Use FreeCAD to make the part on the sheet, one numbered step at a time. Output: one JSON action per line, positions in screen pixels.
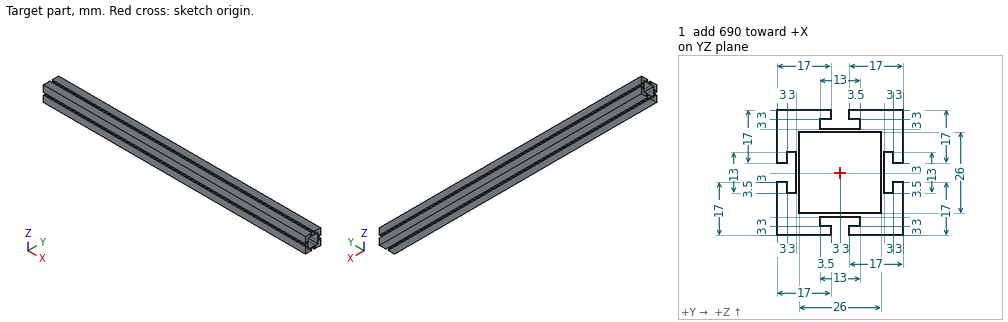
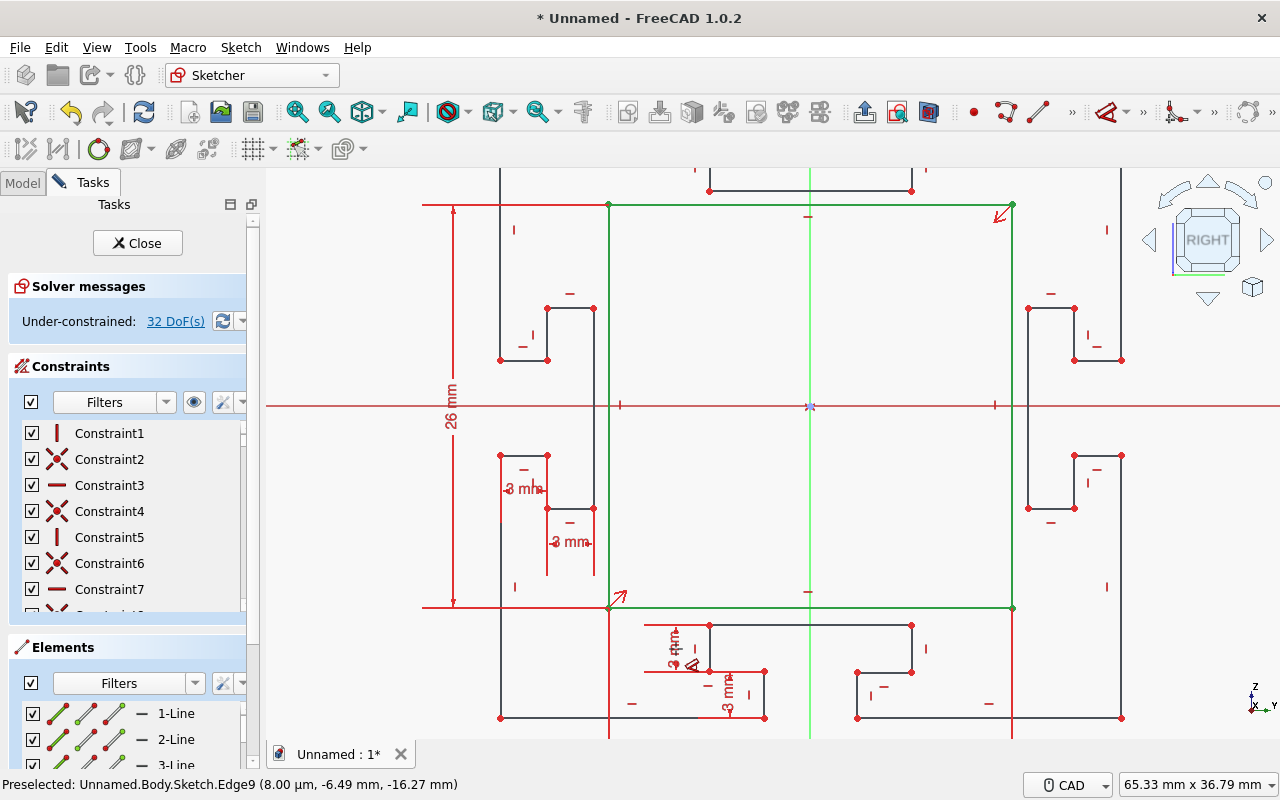
{"action": "left_click", "coordinate": [912, 639]}
{"action": "left_click", "coordinate": [946, 649]}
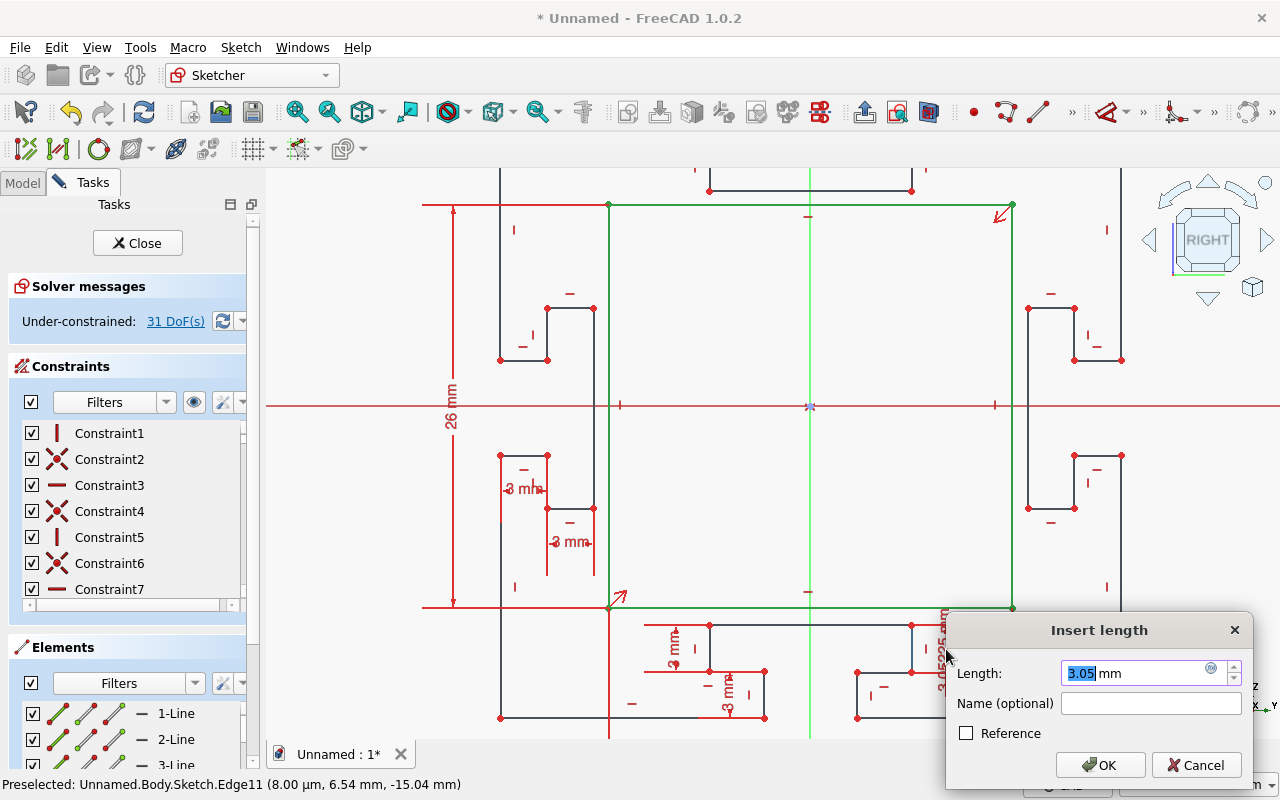
{"action": "type", "text": "3"}
{"action": "key", "text": "Return"}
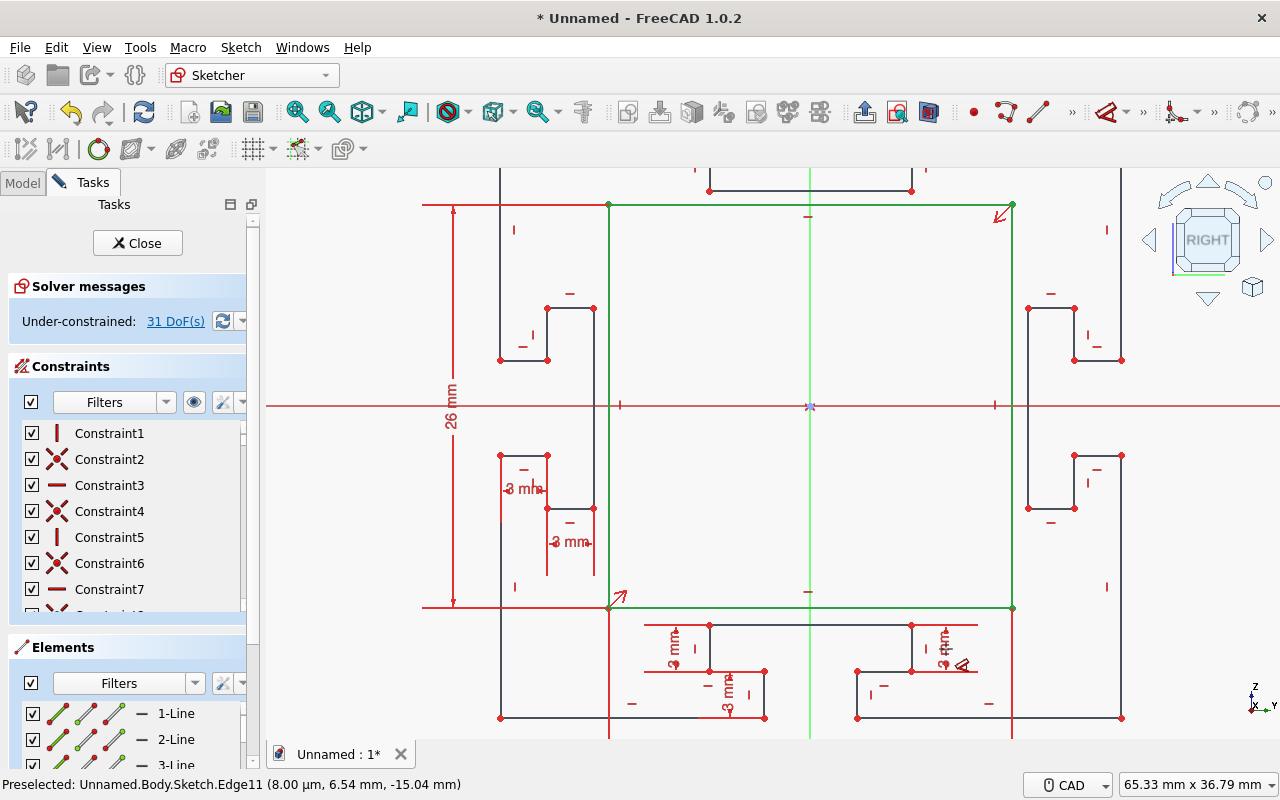
{"action": "left_click", "coordinate": [857, 686]}
{"action": "left_click", "coordinate": [891, 691]}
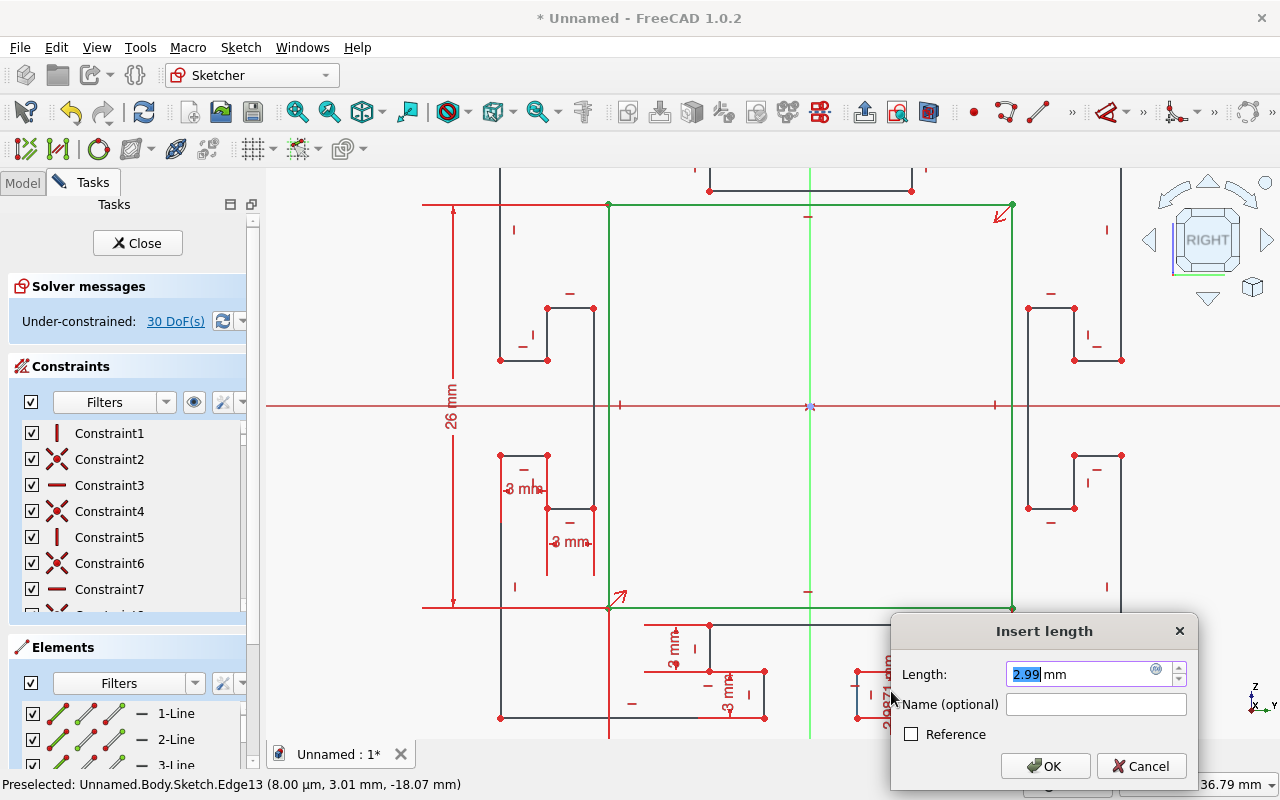
{"action": "type", "text": "3"}
{"action": "key", "text": "Return"}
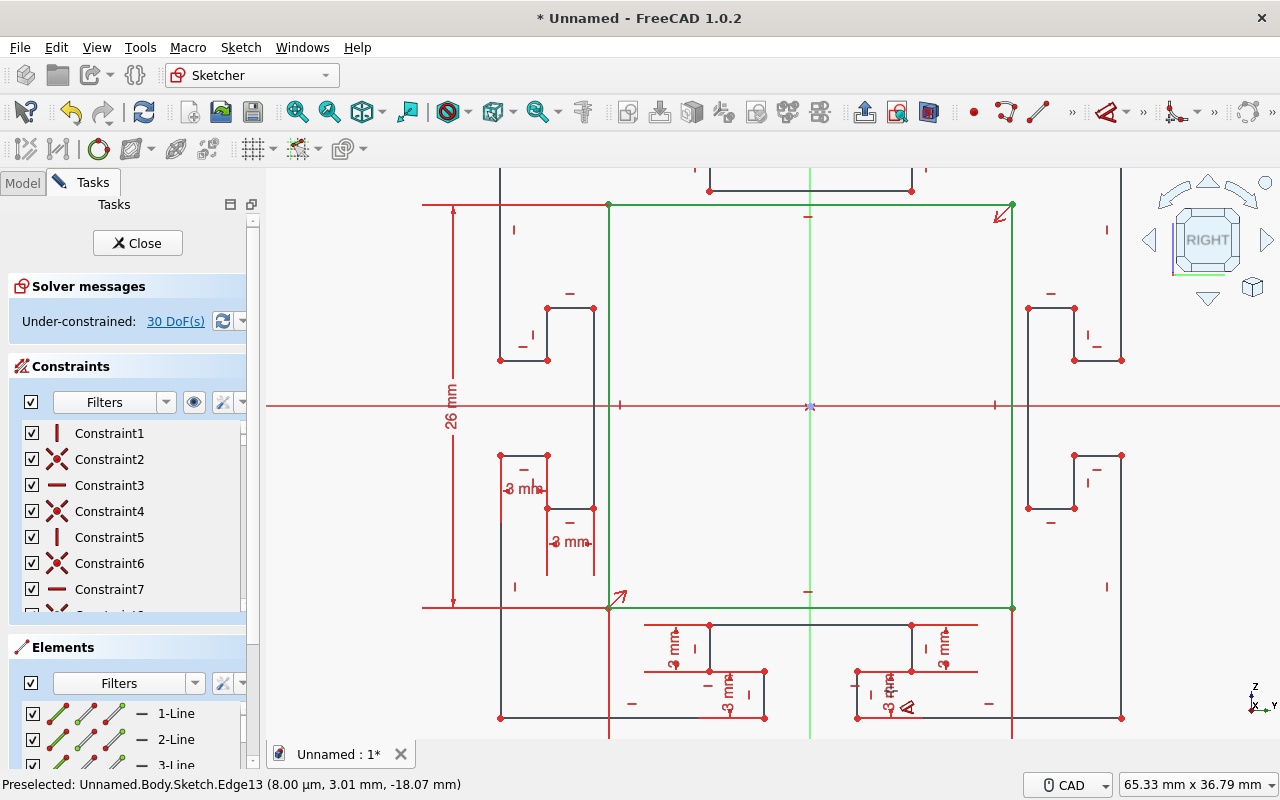
{"action": "left_click", "coordinate": [1107, 456]}
{"action": "left_click", "coordinate": [1095, 490]}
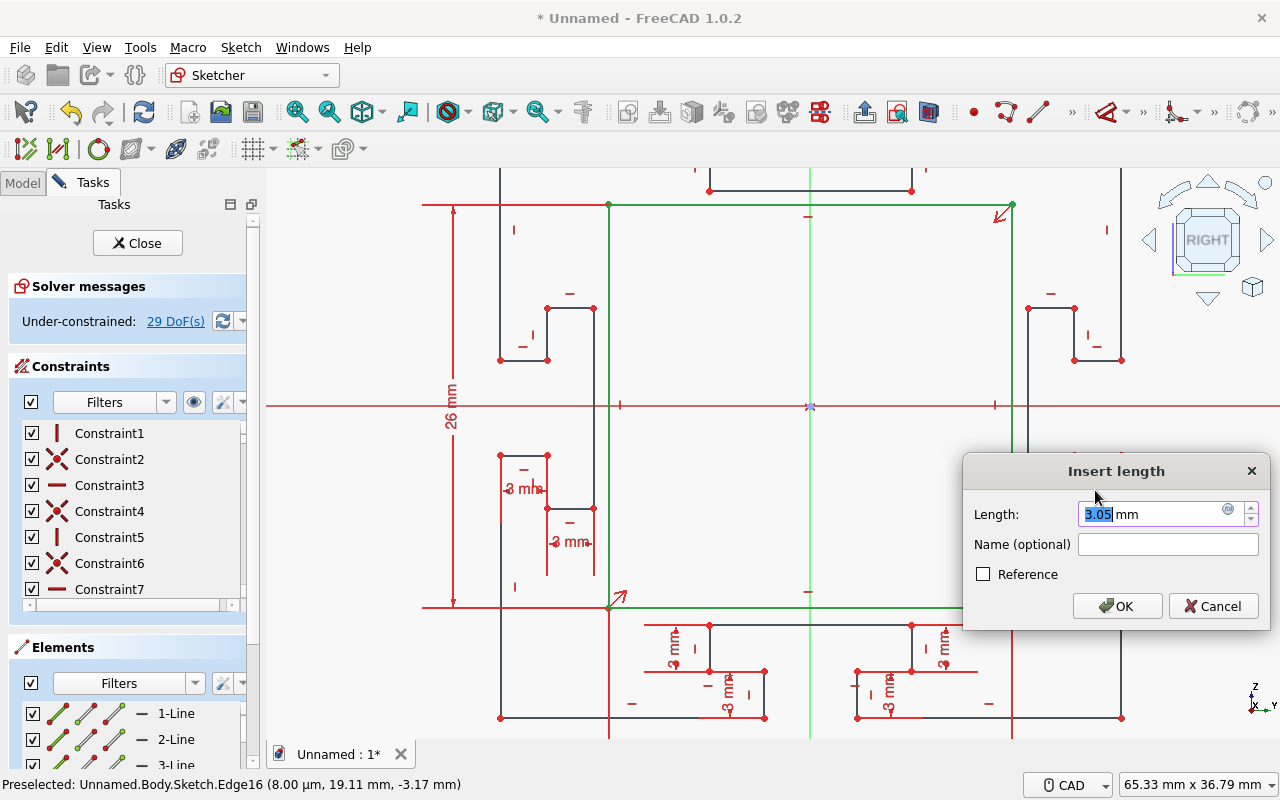
{"action": "type", "text": "3"}
{"action": "key", "text": "Return"}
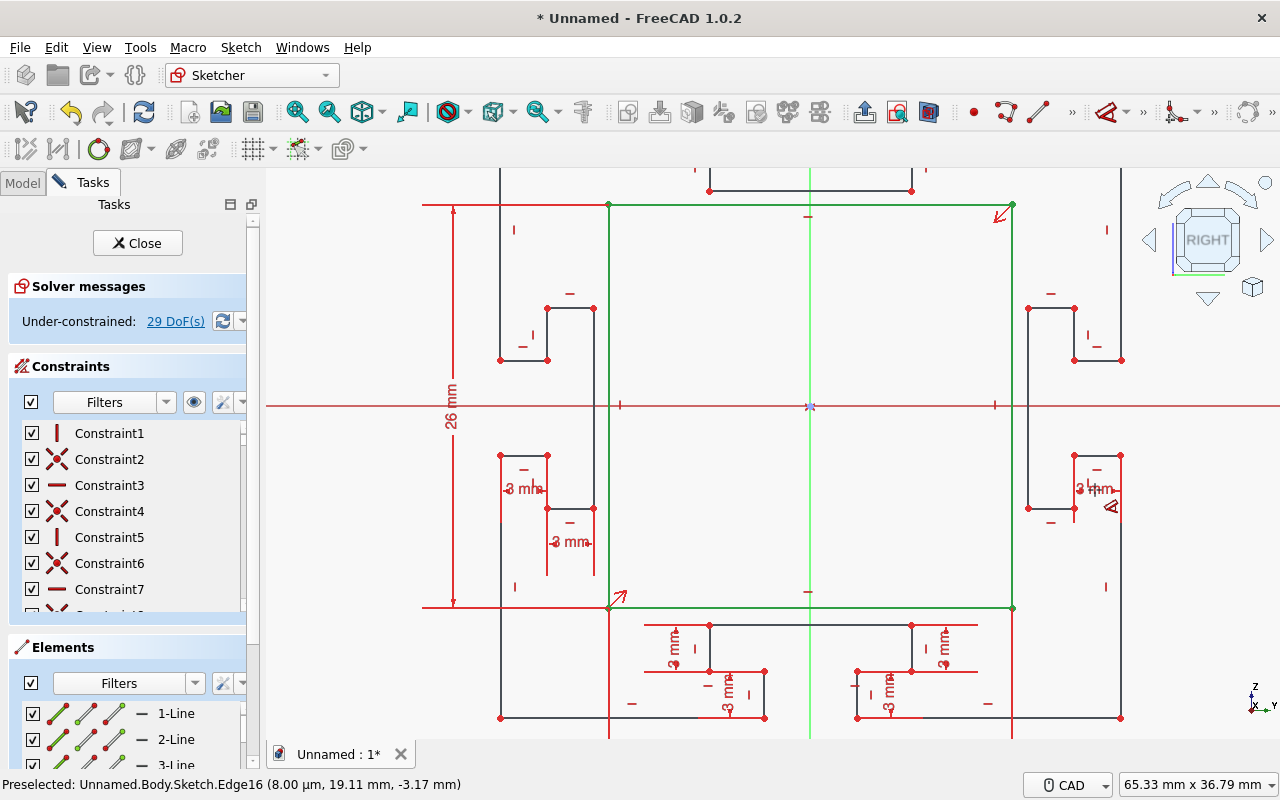
{"action": "left_click", "coordinate": [1060, 509]}
{"action": "left_click", "coordinate": [1051, 543]}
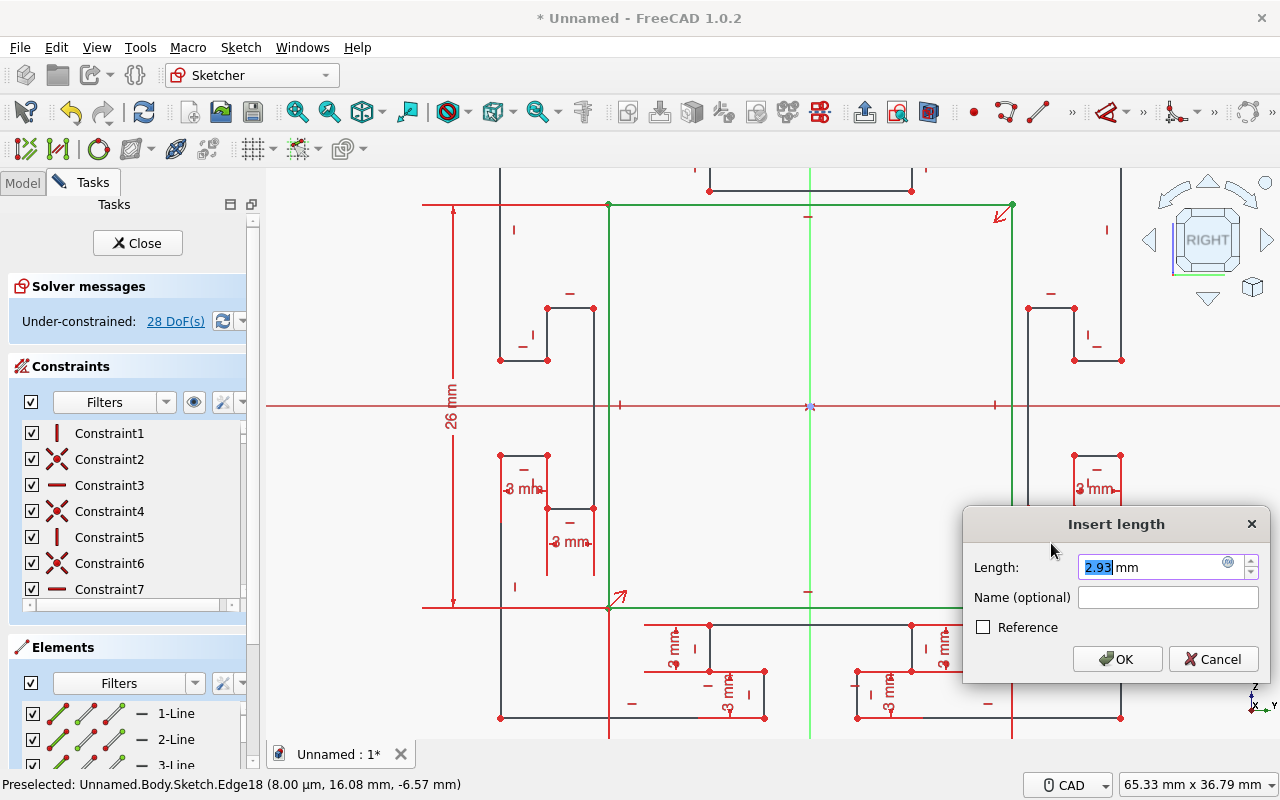
{"action": "type", "text": "3"}
{"action": "key", "text": "Return"}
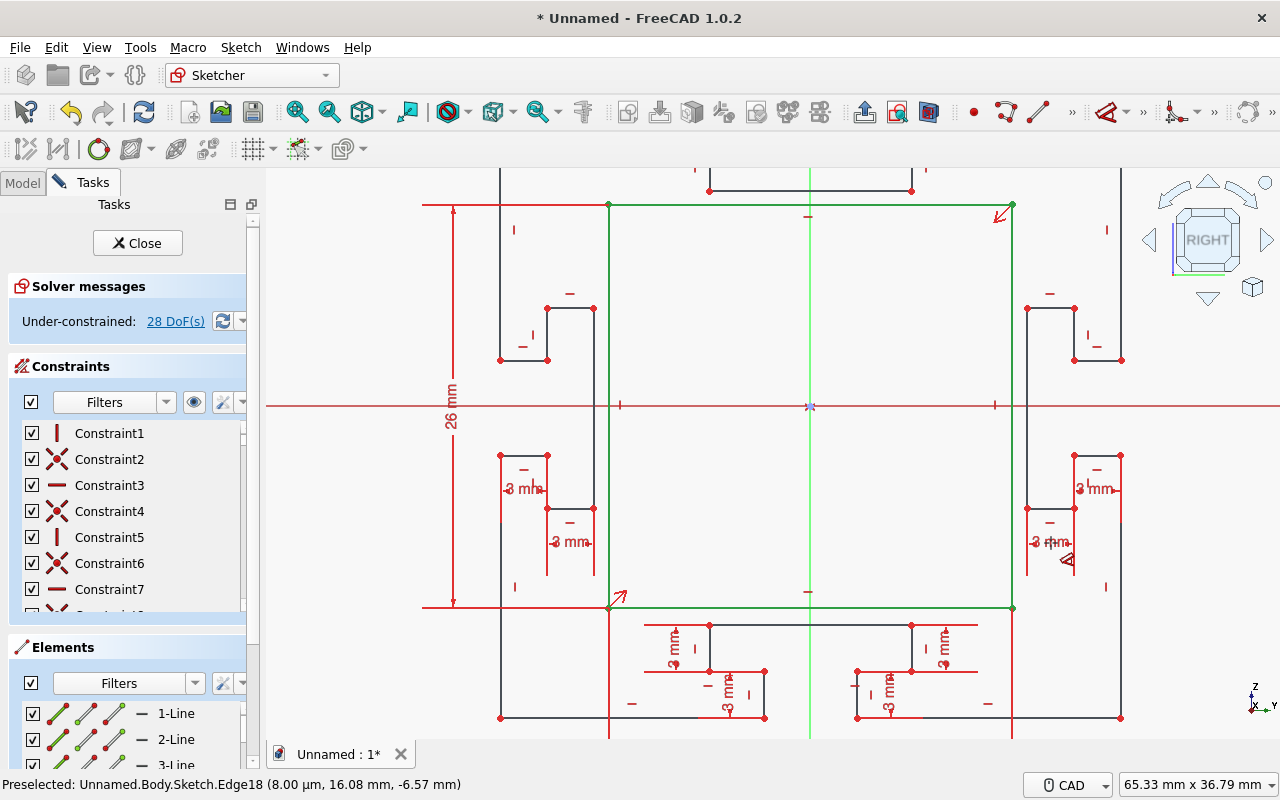
{"action": "left_click", "coordinate": [1041, 308]}
{"action": "left_click", "coordinate": [1051, 274]}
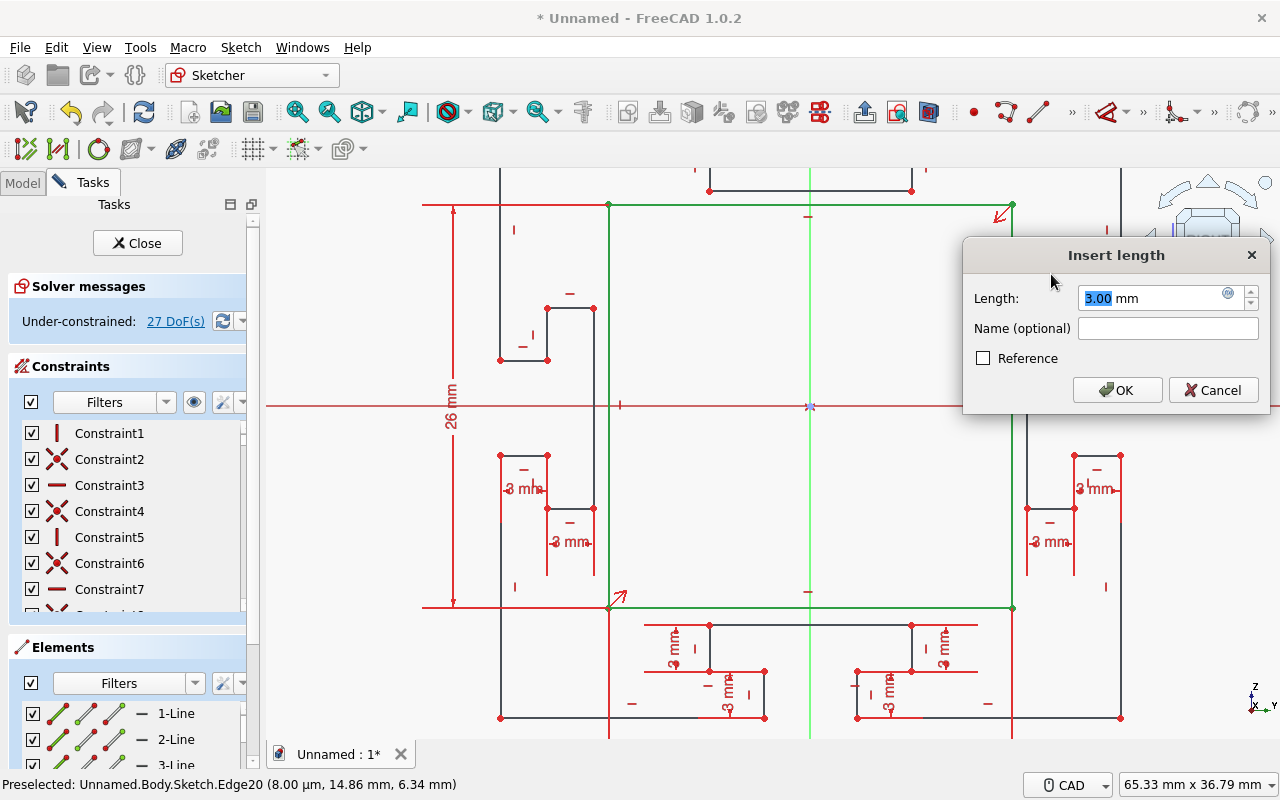
{"action": "type", "text": "3"}
{"action": "key", "text": "Return"}